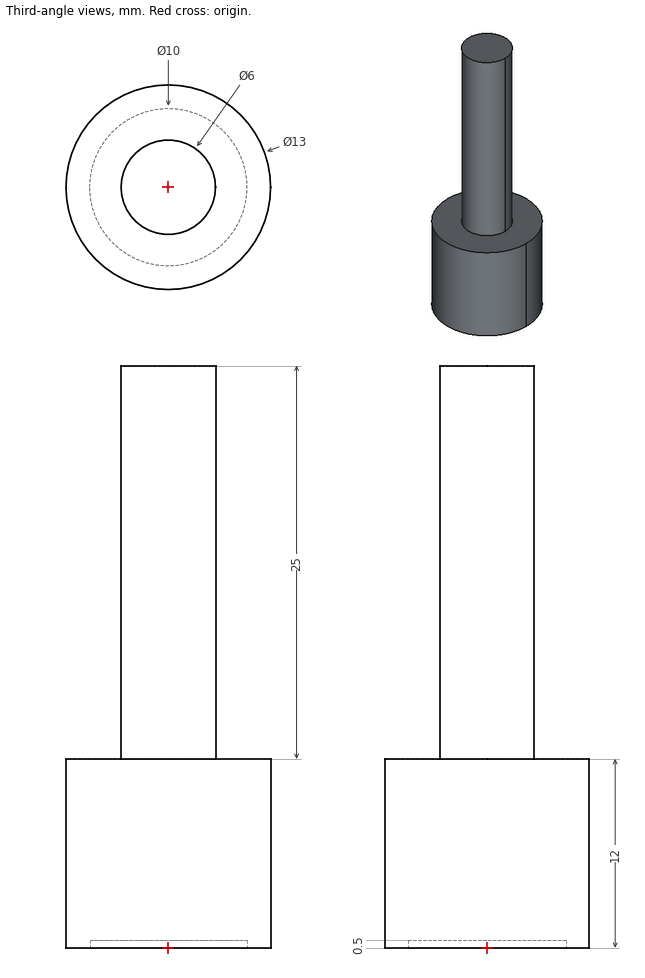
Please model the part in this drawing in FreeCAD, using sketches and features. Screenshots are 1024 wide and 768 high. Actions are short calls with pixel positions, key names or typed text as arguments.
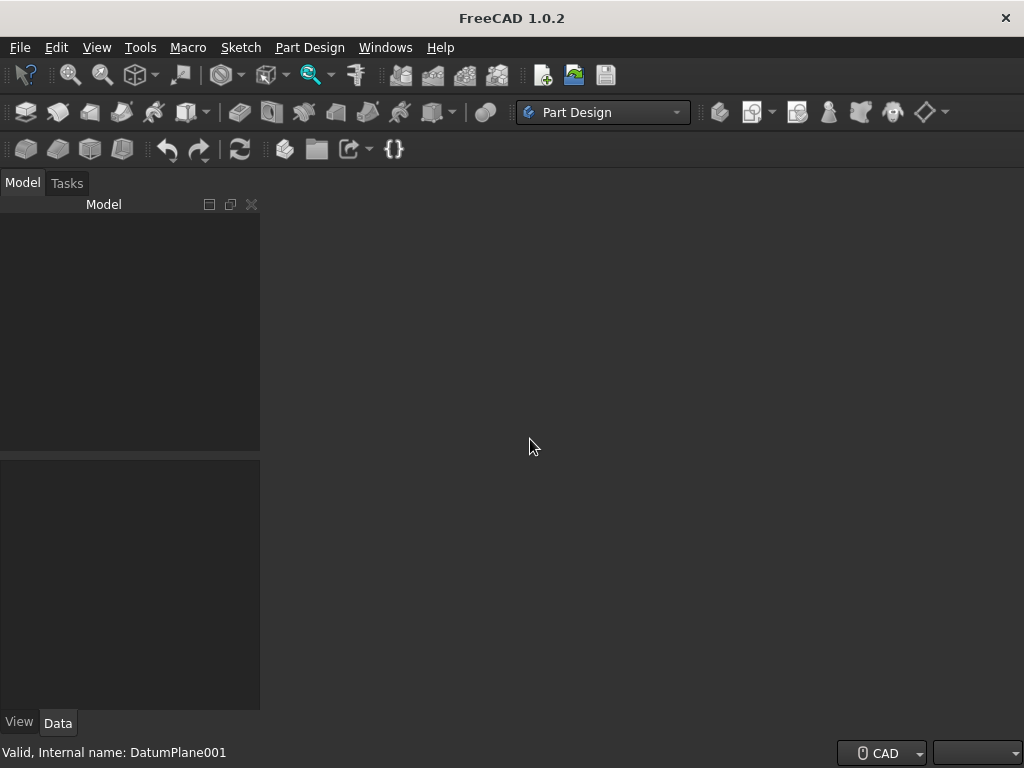
click(542, 76)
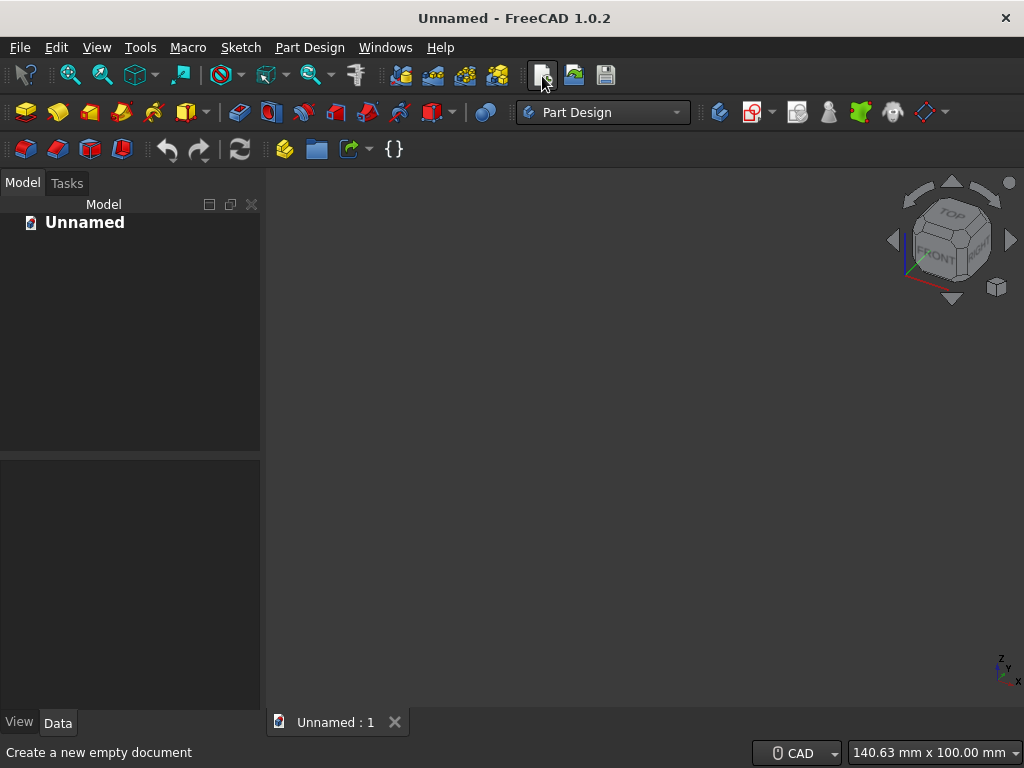
click(752, 112)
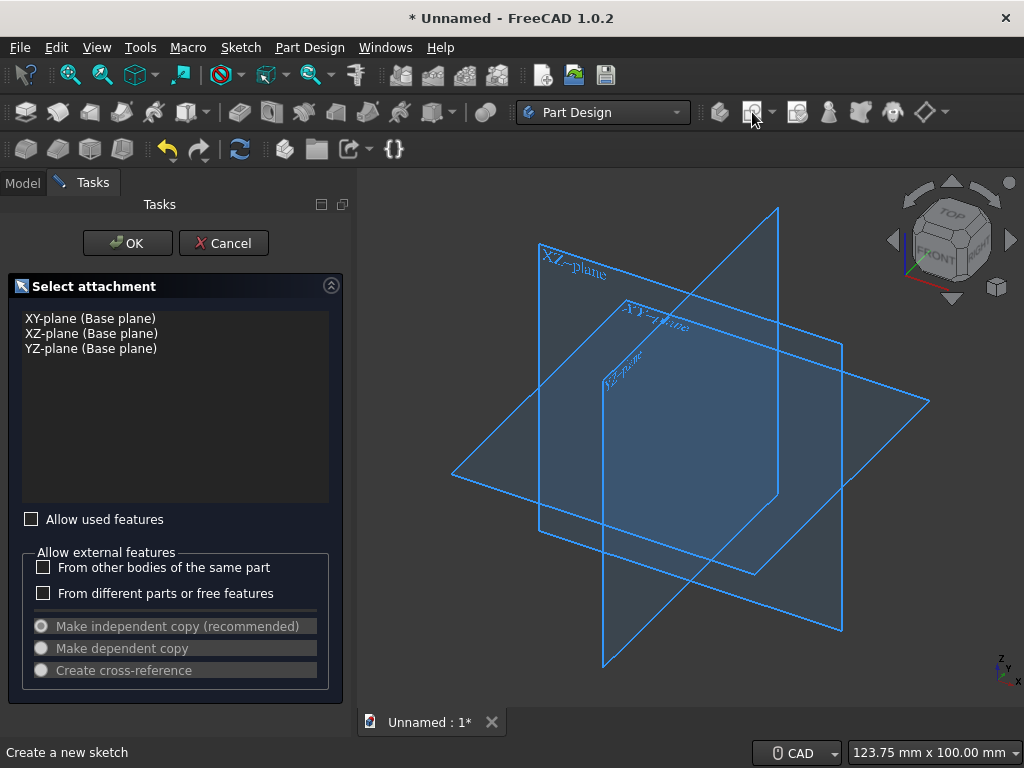
click(82, 318)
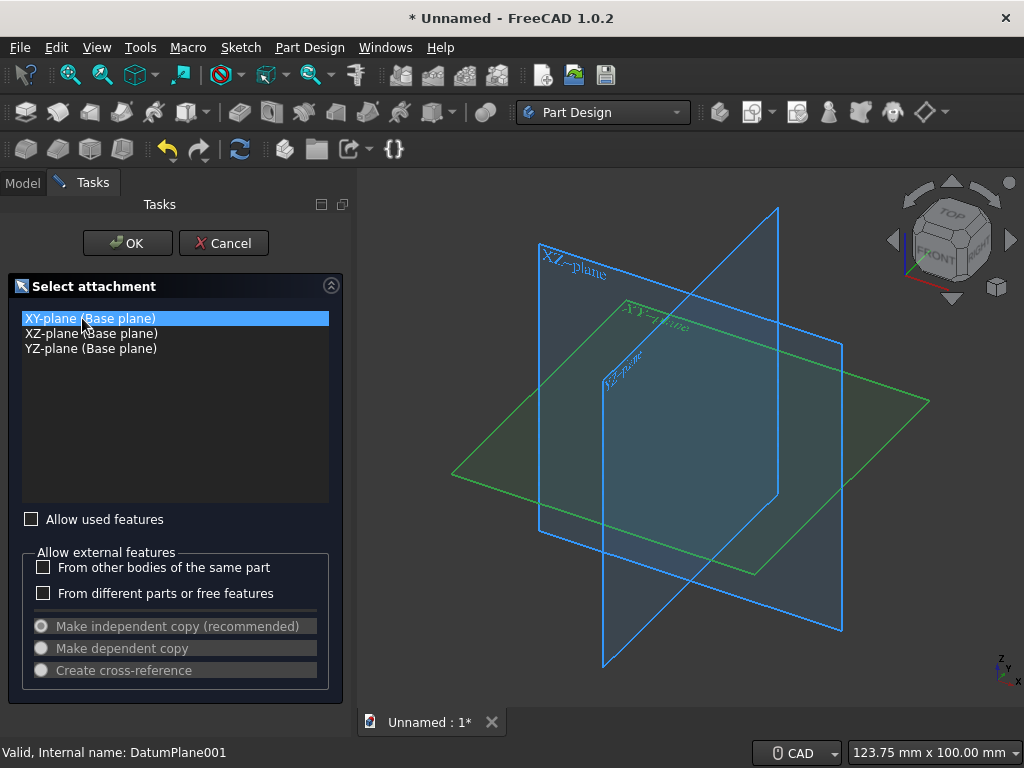
click(128, 243)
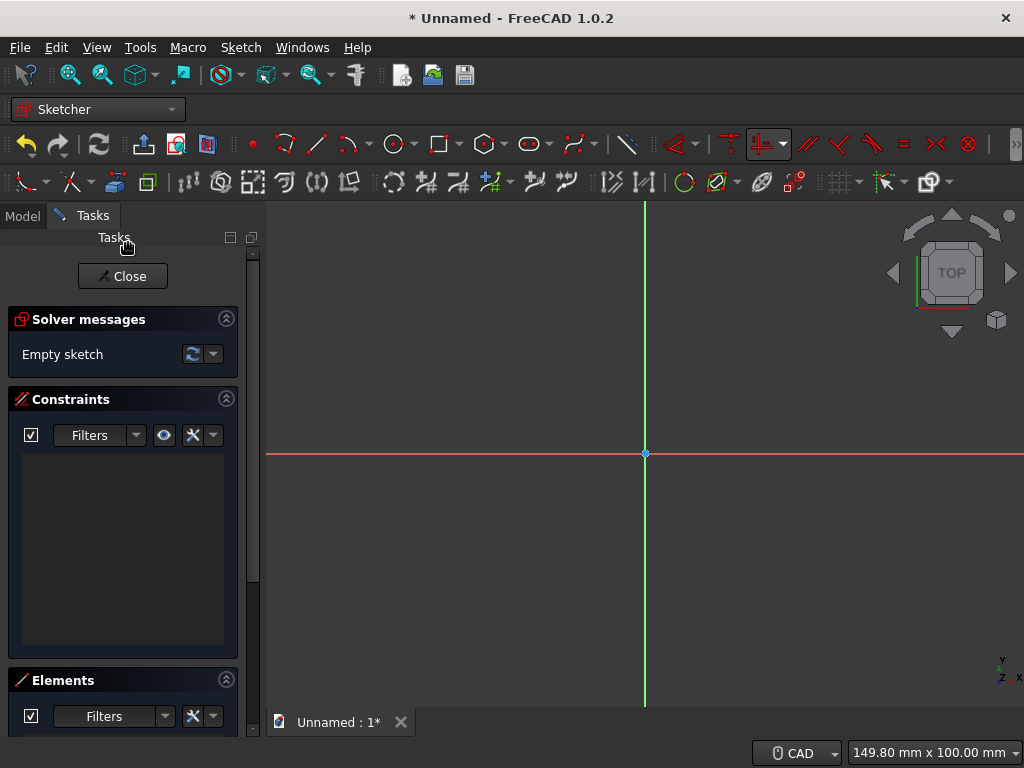
scroll(662, 454, up, 8)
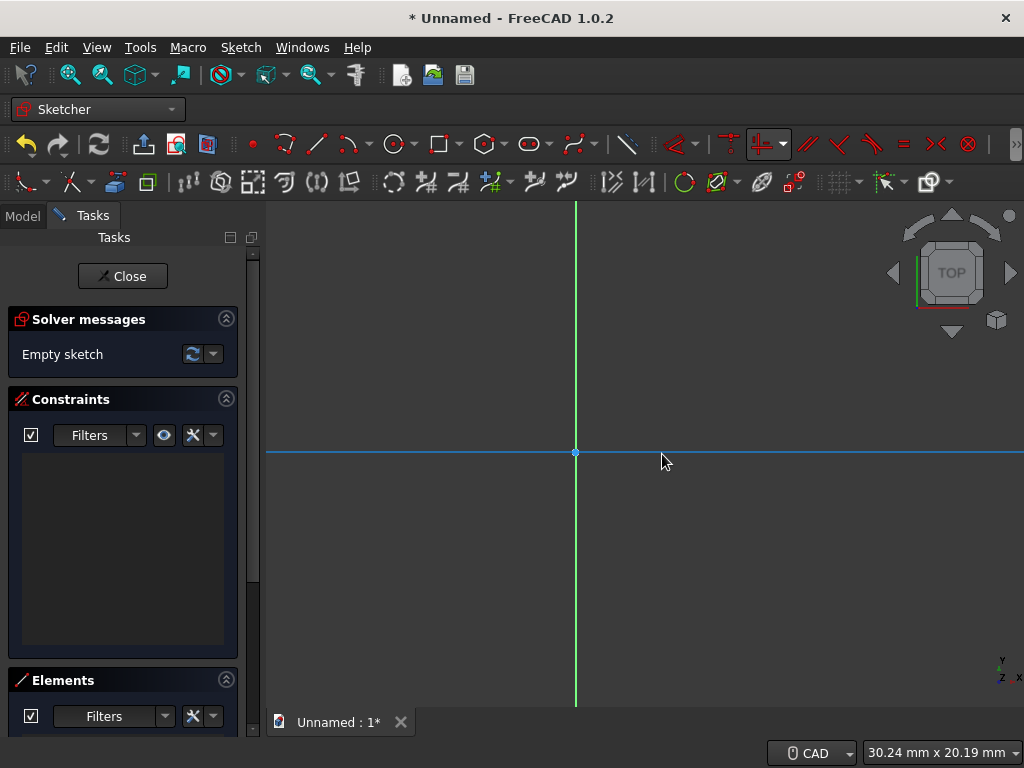
click(394, 144)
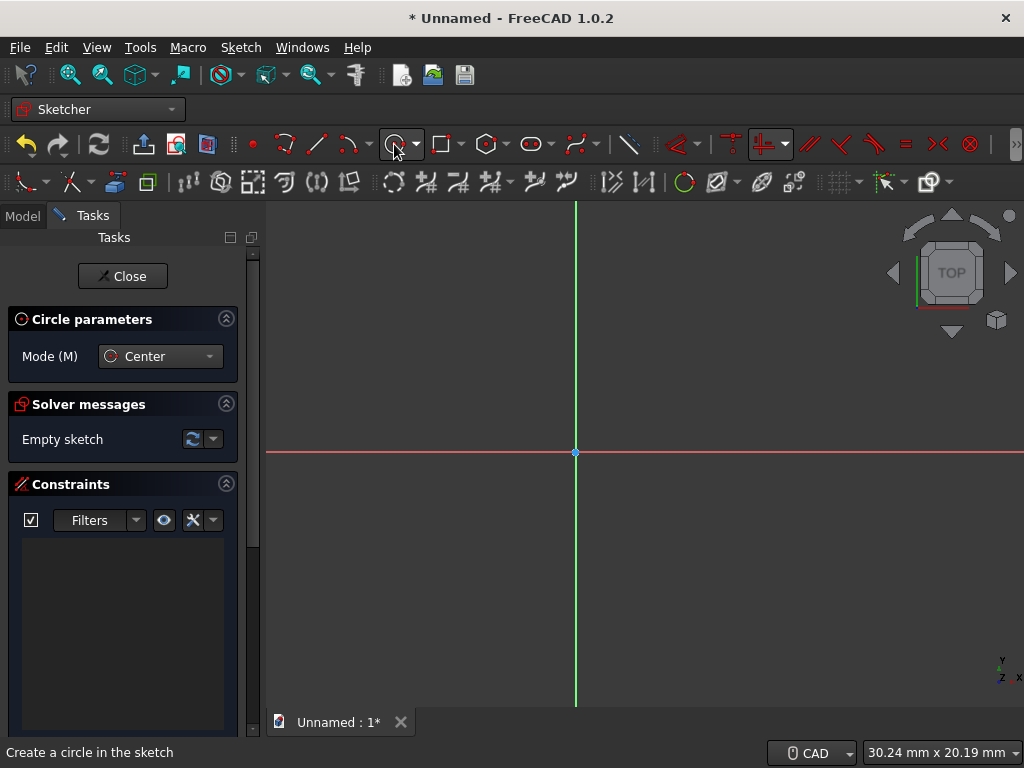
click(576, 452)
move(691, 337)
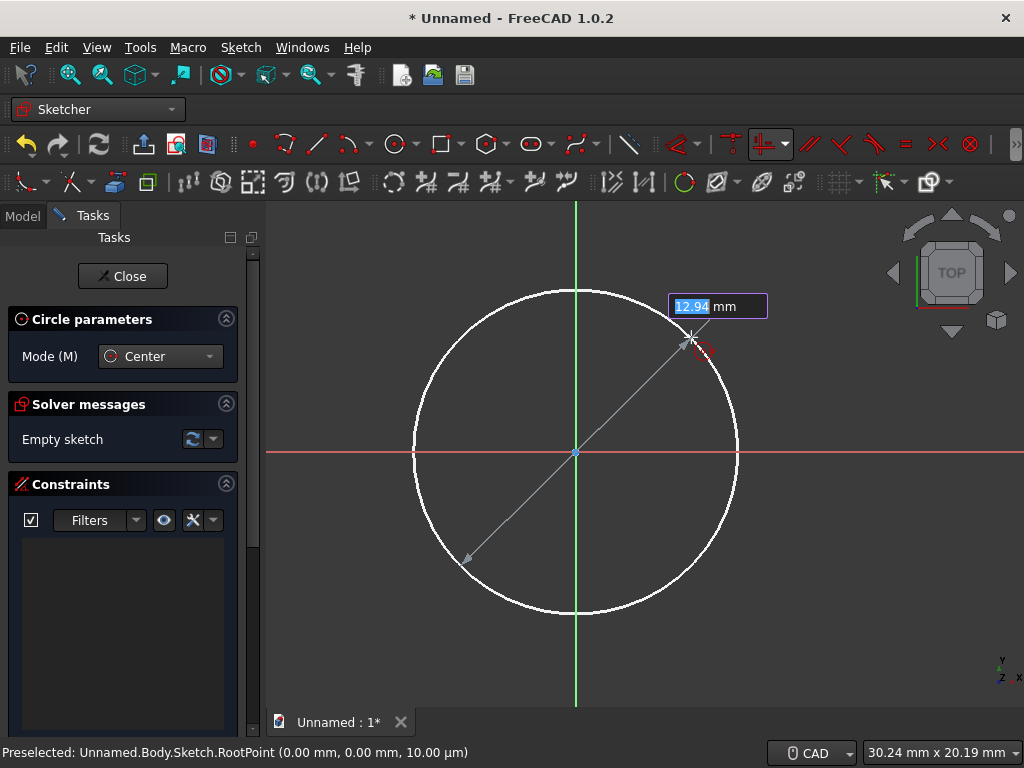
text(13)
key(Return)
key(Escape)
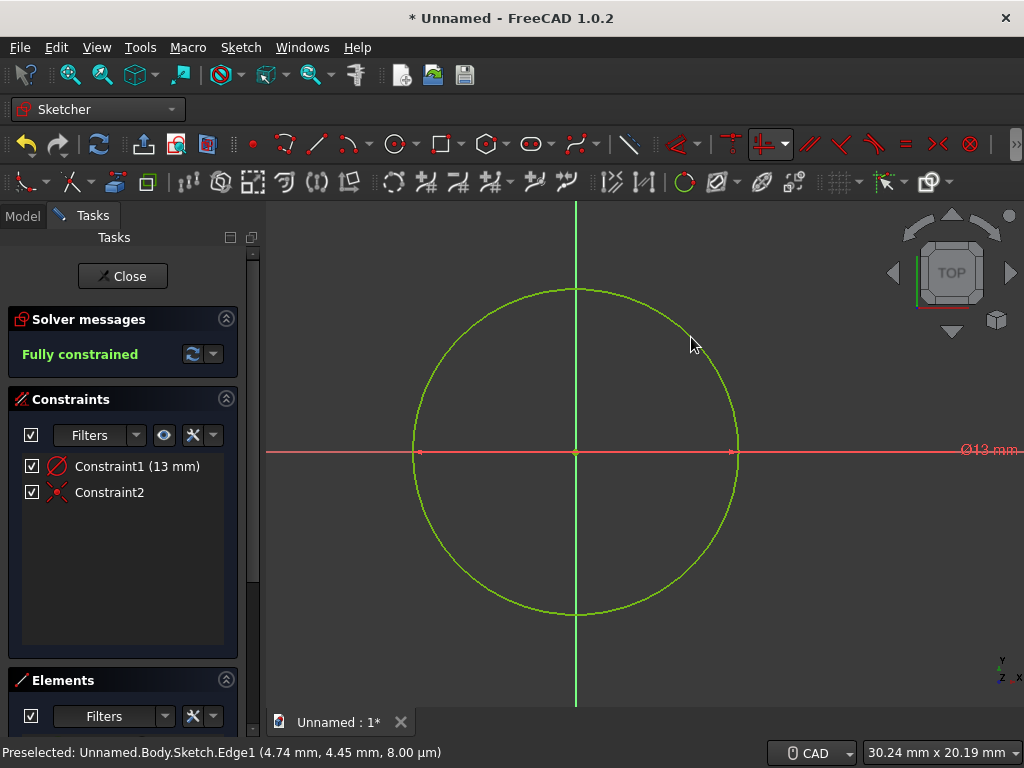
click(123, 276)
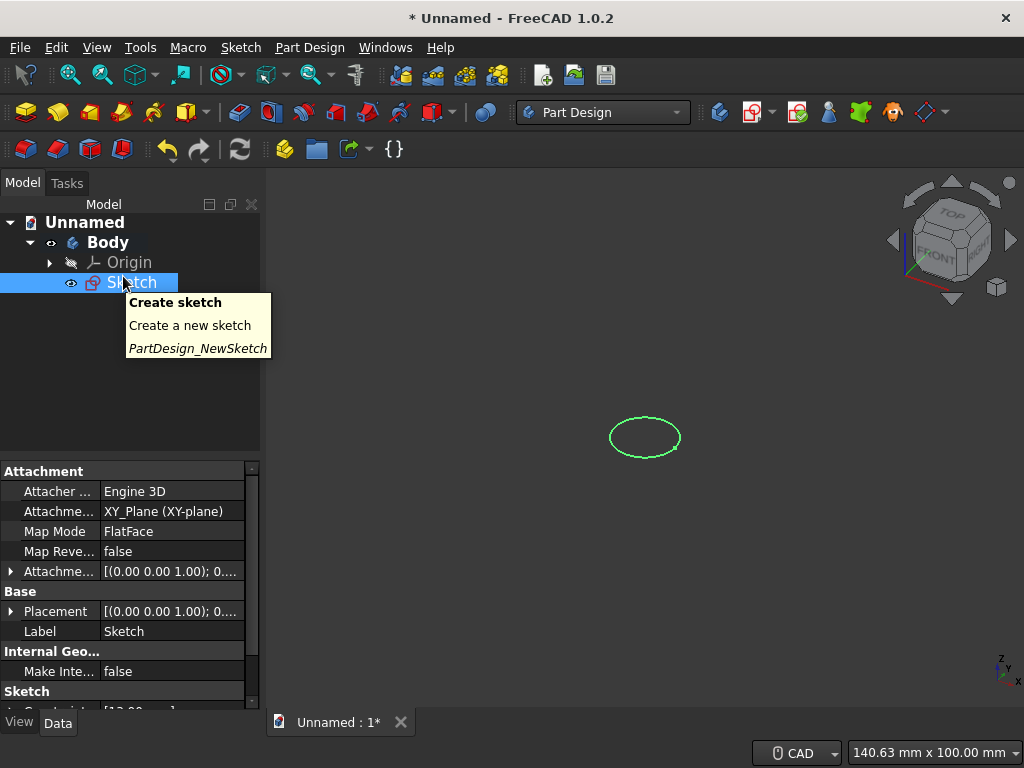
click(26, 112)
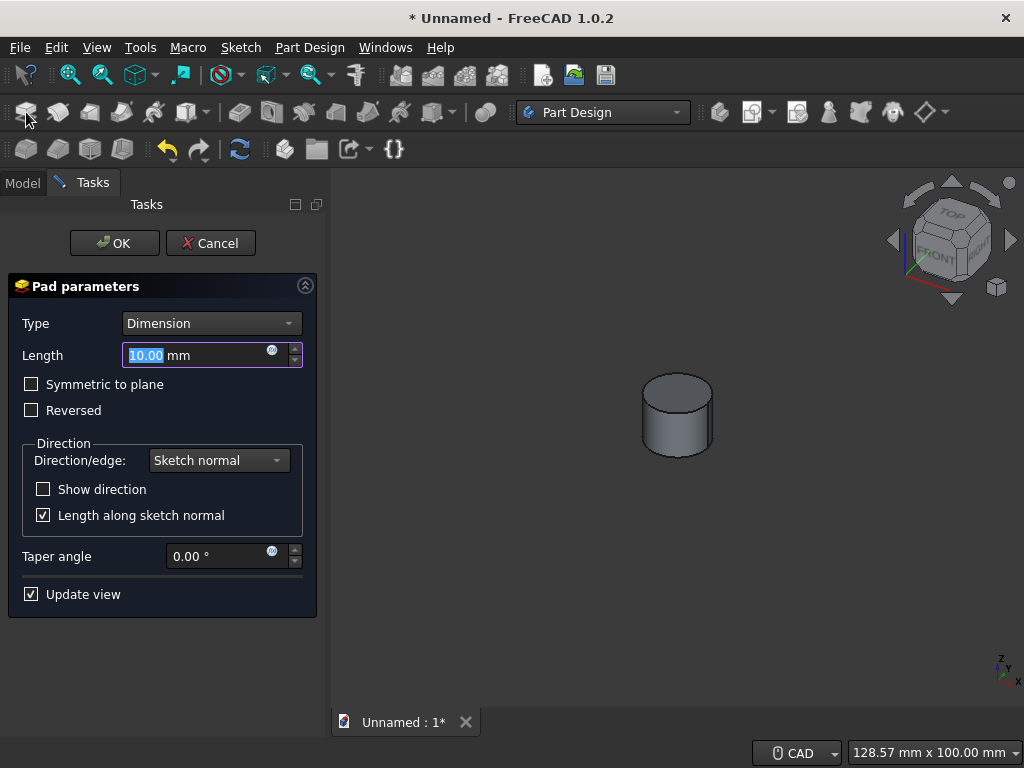
text(12)
key(Tab)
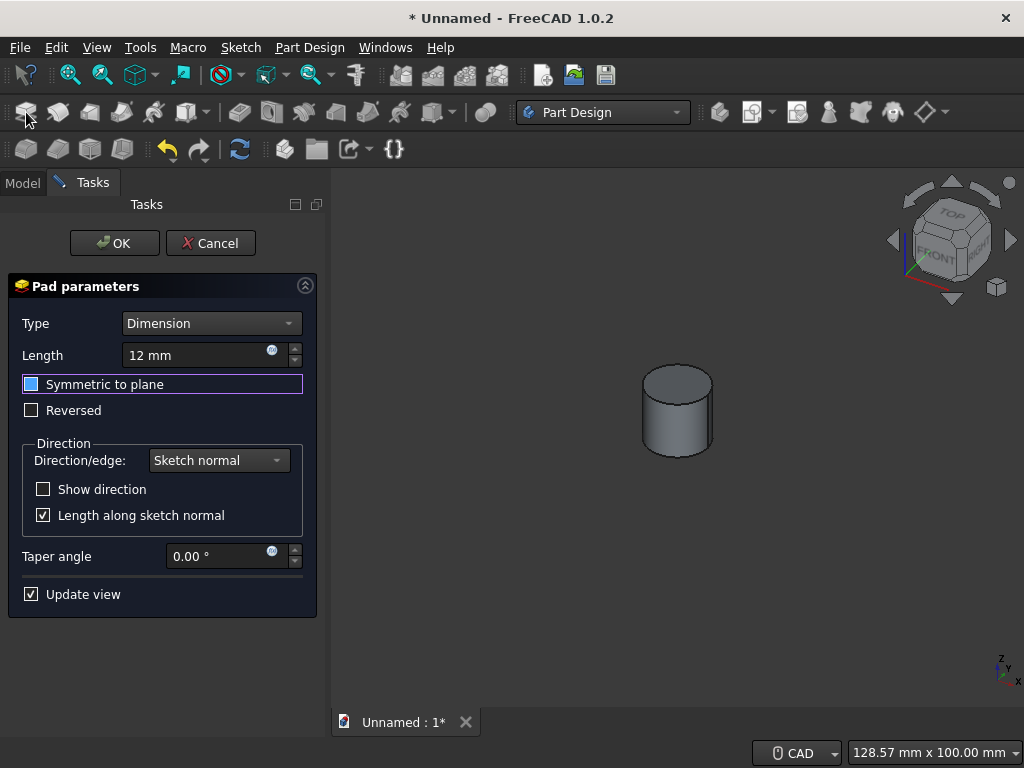
click(115, 243)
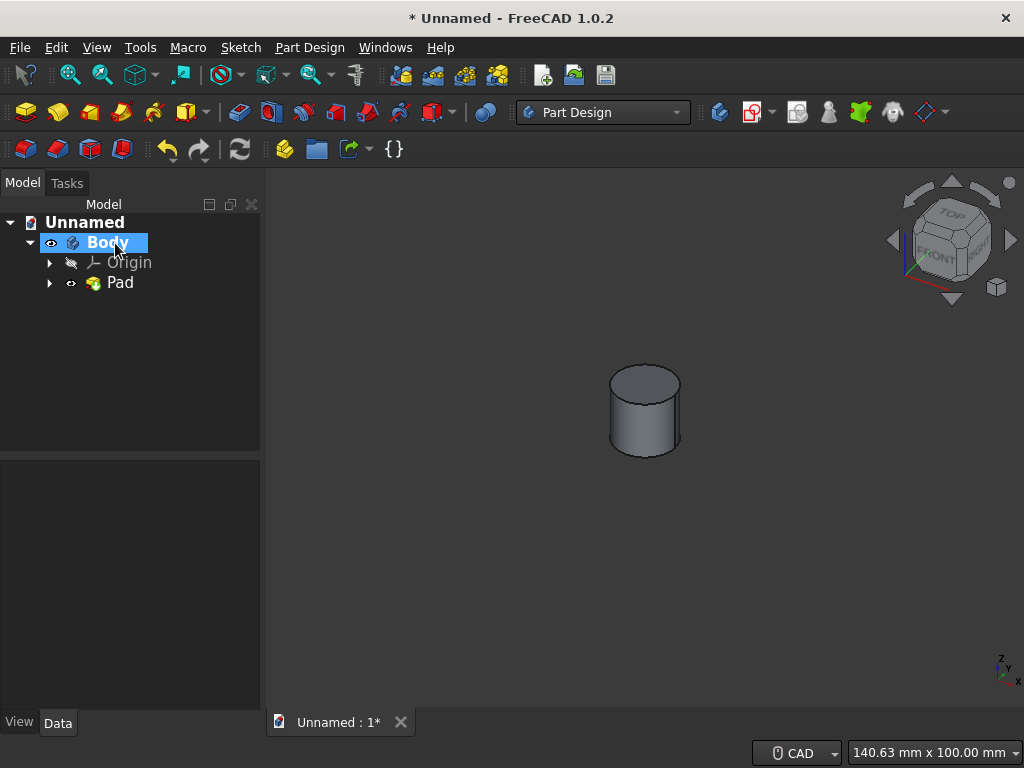
click(72, 76)